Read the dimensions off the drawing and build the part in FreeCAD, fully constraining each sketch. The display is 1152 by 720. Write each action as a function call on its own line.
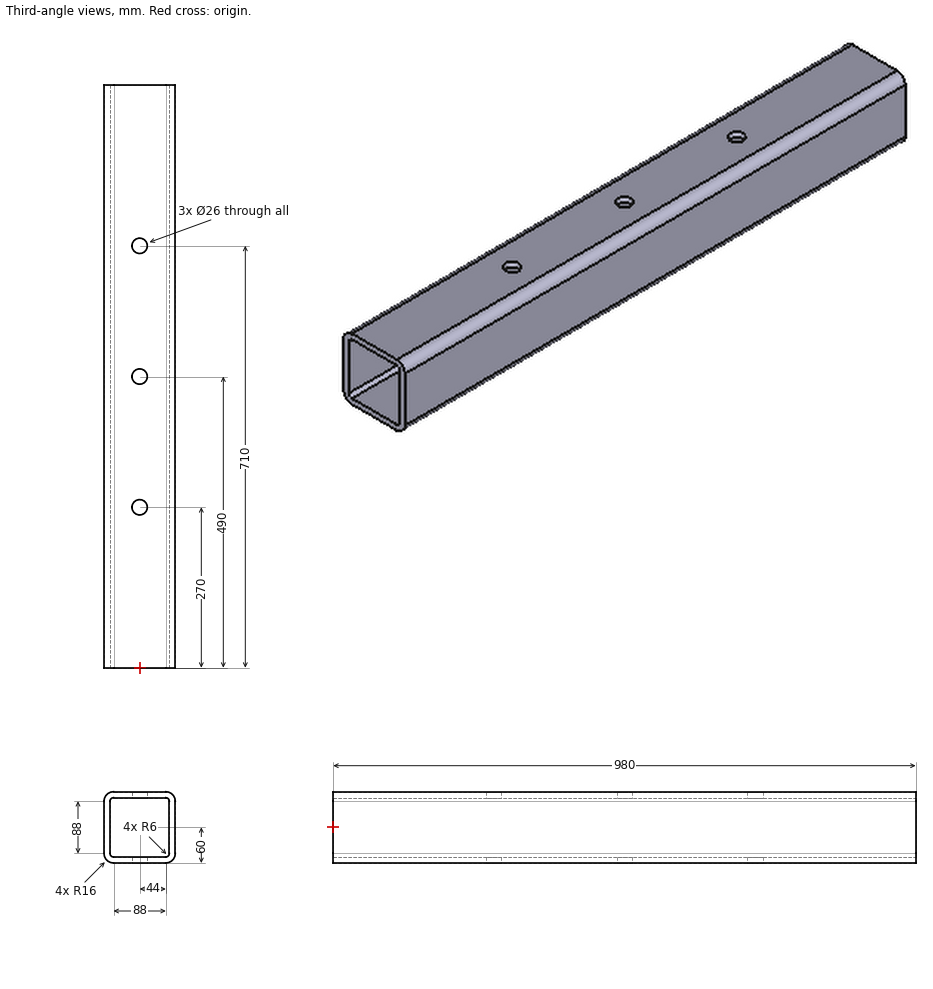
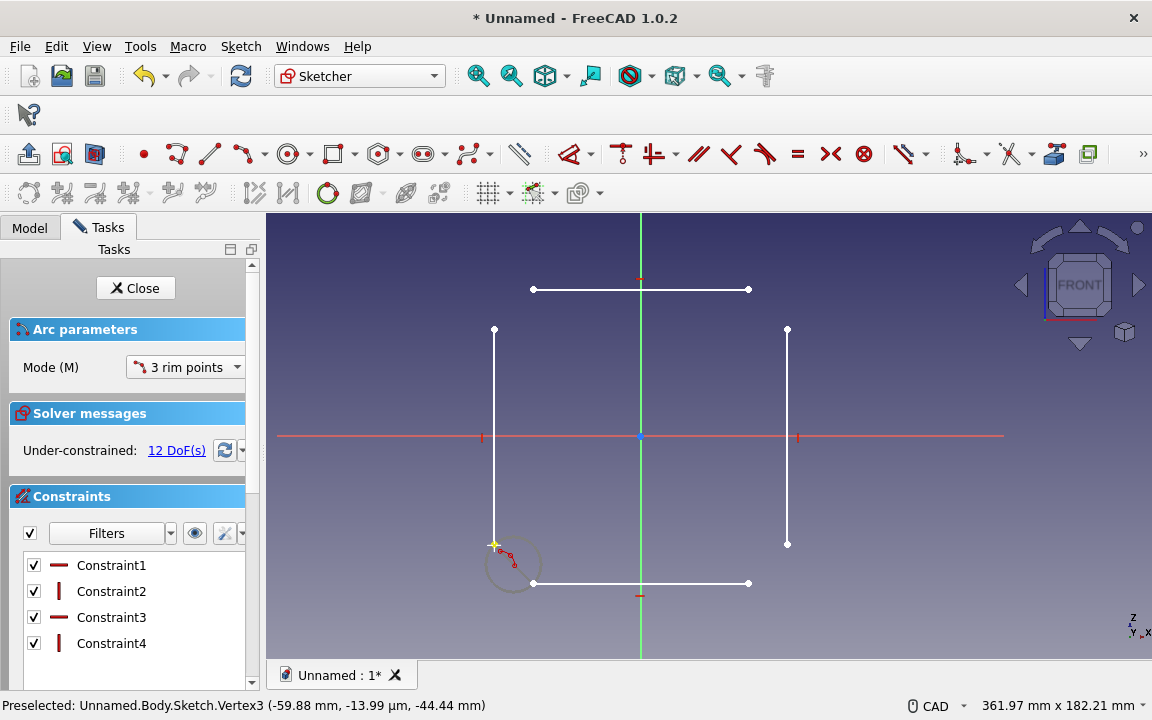
scroll(505, 572, up, 2)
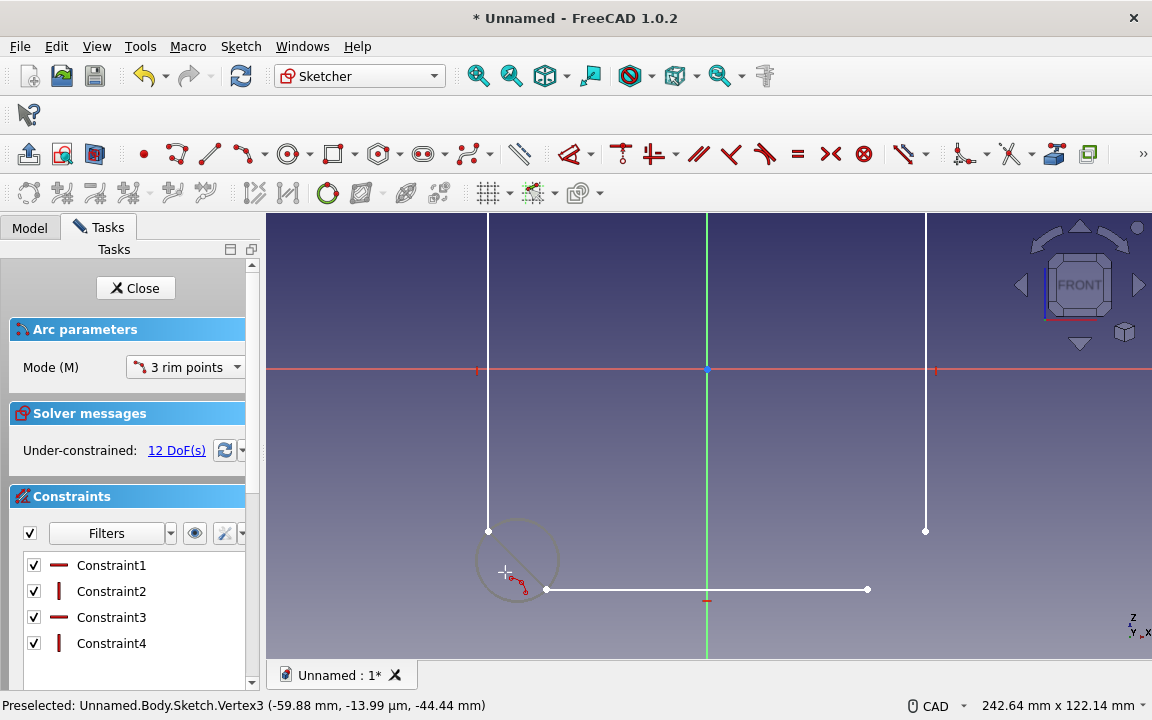
click(505, 571)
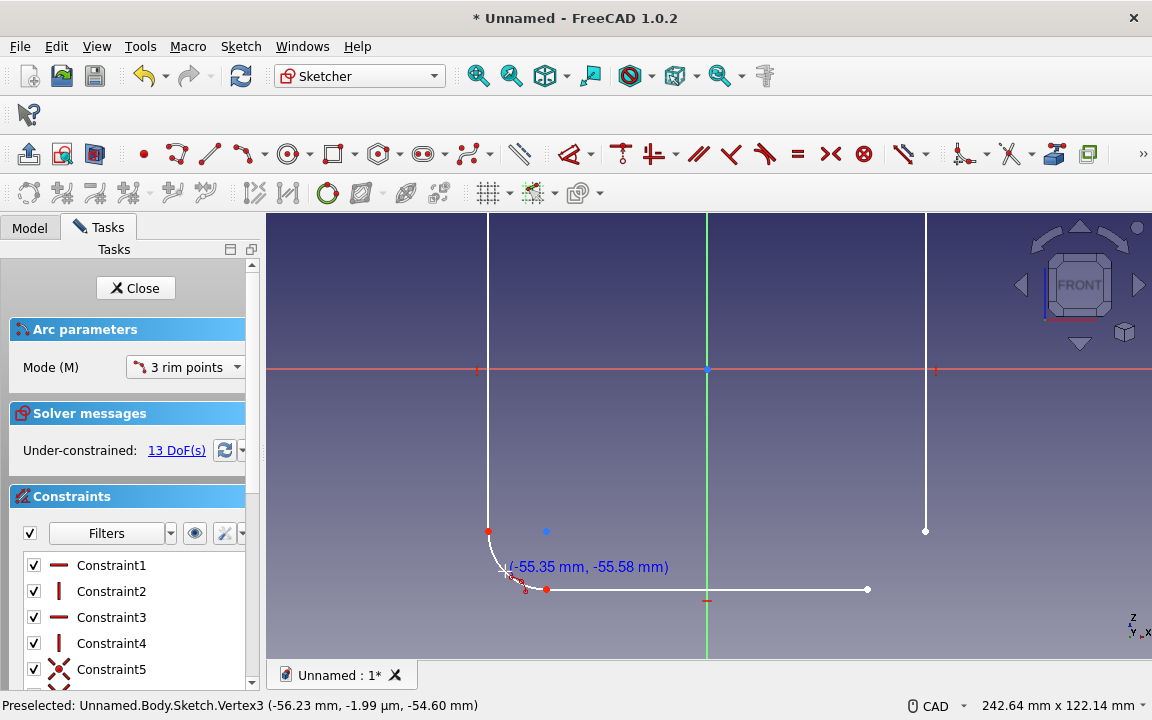
scroll(505, 572, down, 2)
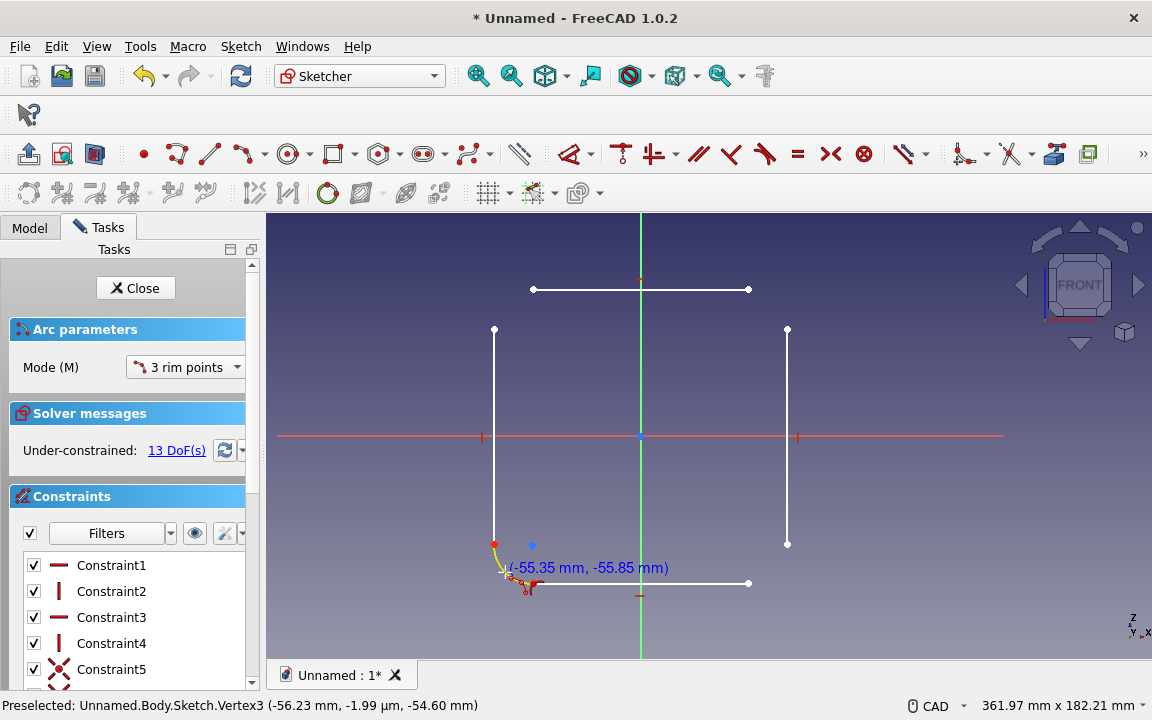
click(494, 330)
click(533, 290)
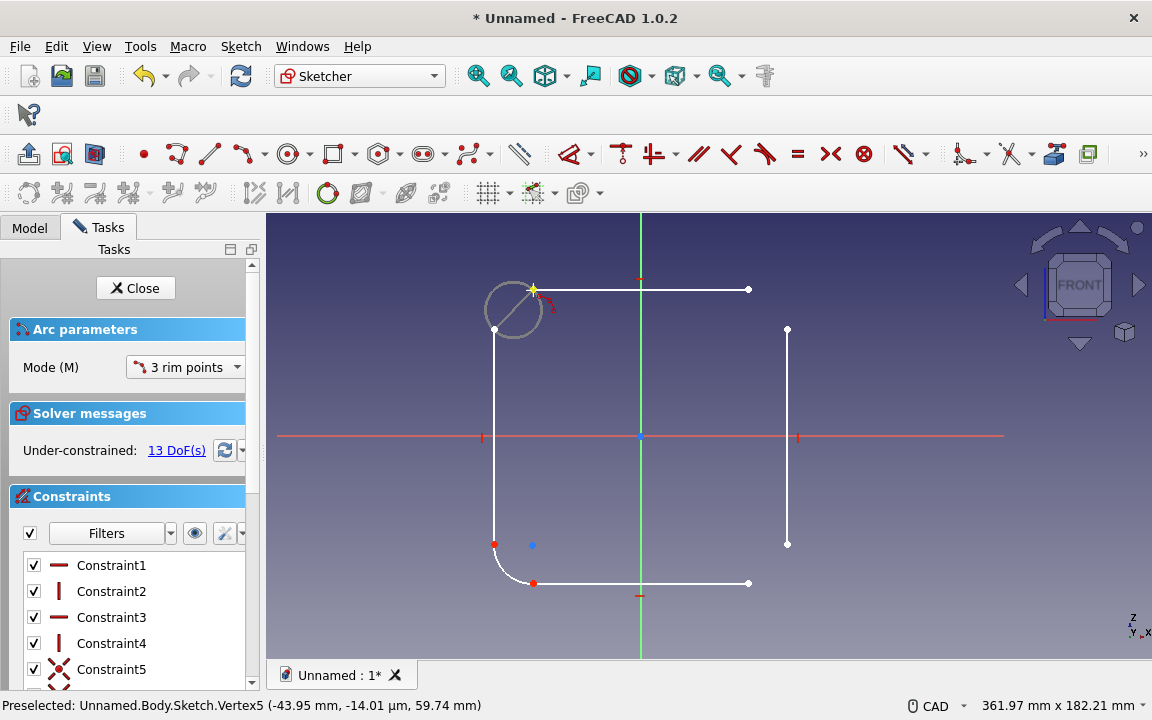
scroll(505, 301, up, 2)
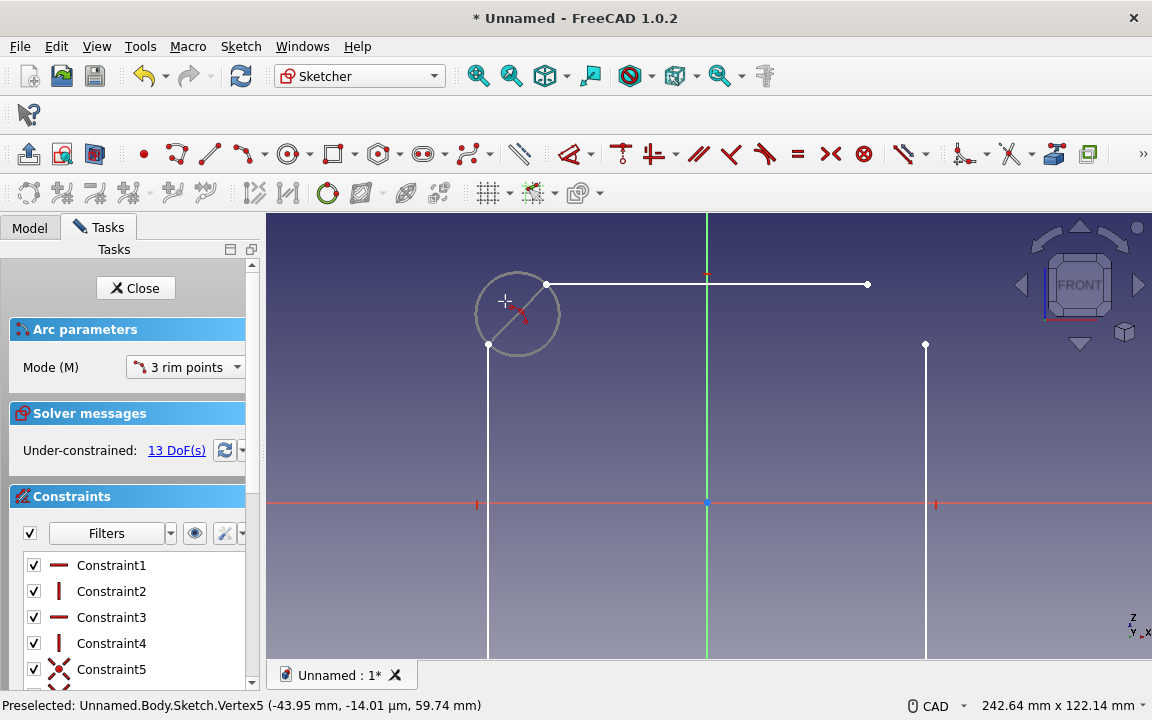
click(505, 301)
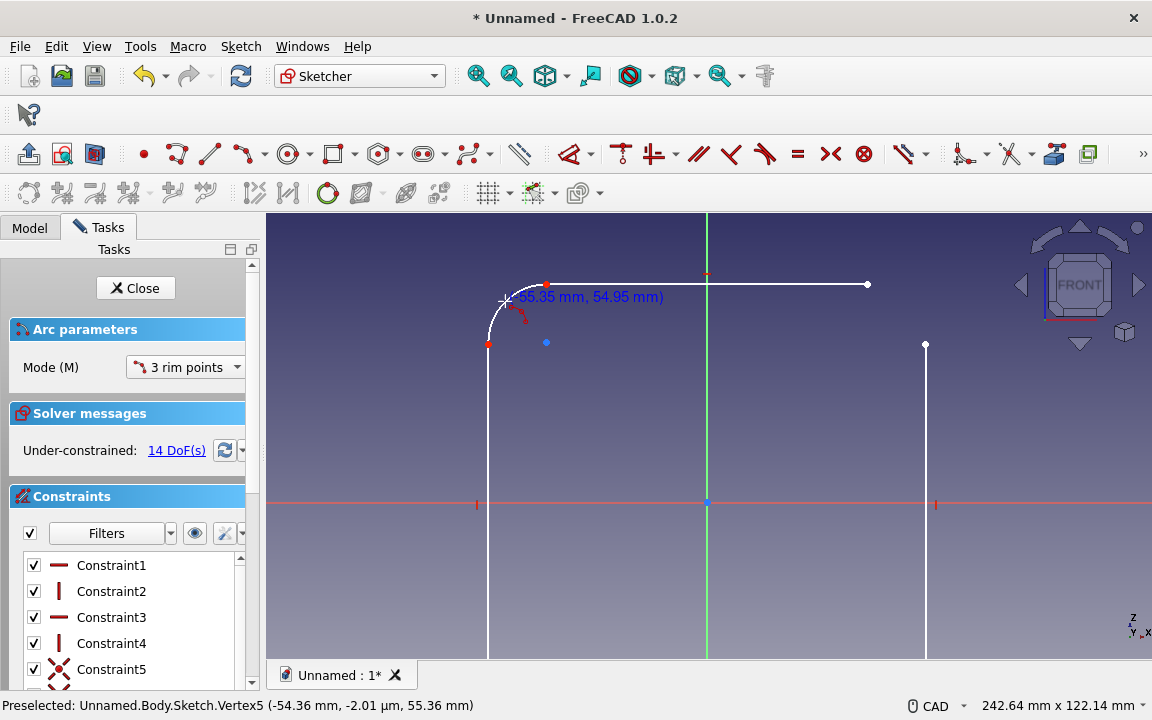
click(867, 284)
click(926, 344)
click(909, 301)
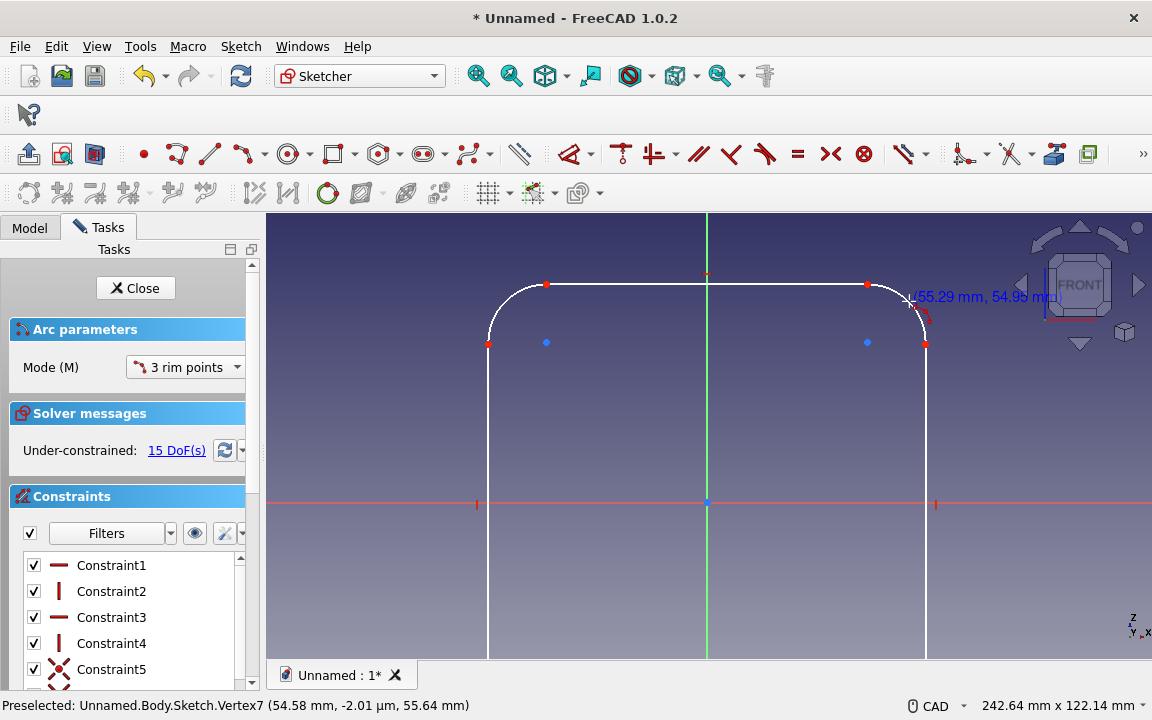
scroll(505, 301, down, 2)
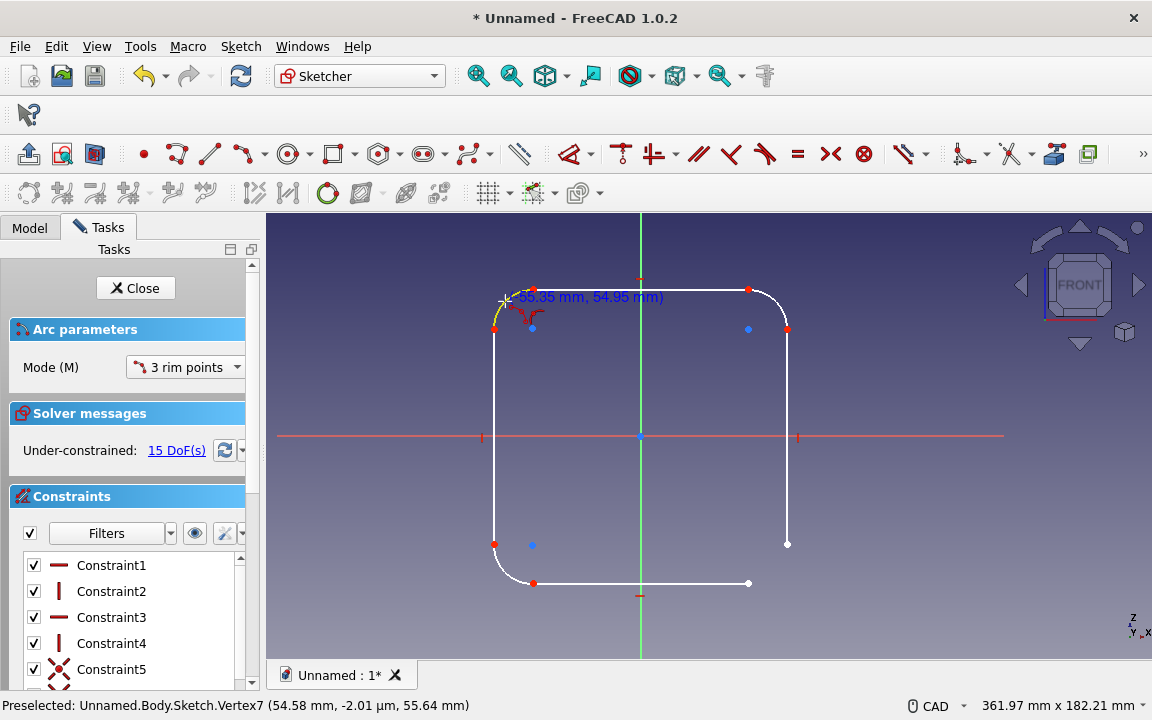
click(787, 545)
click(748, 584)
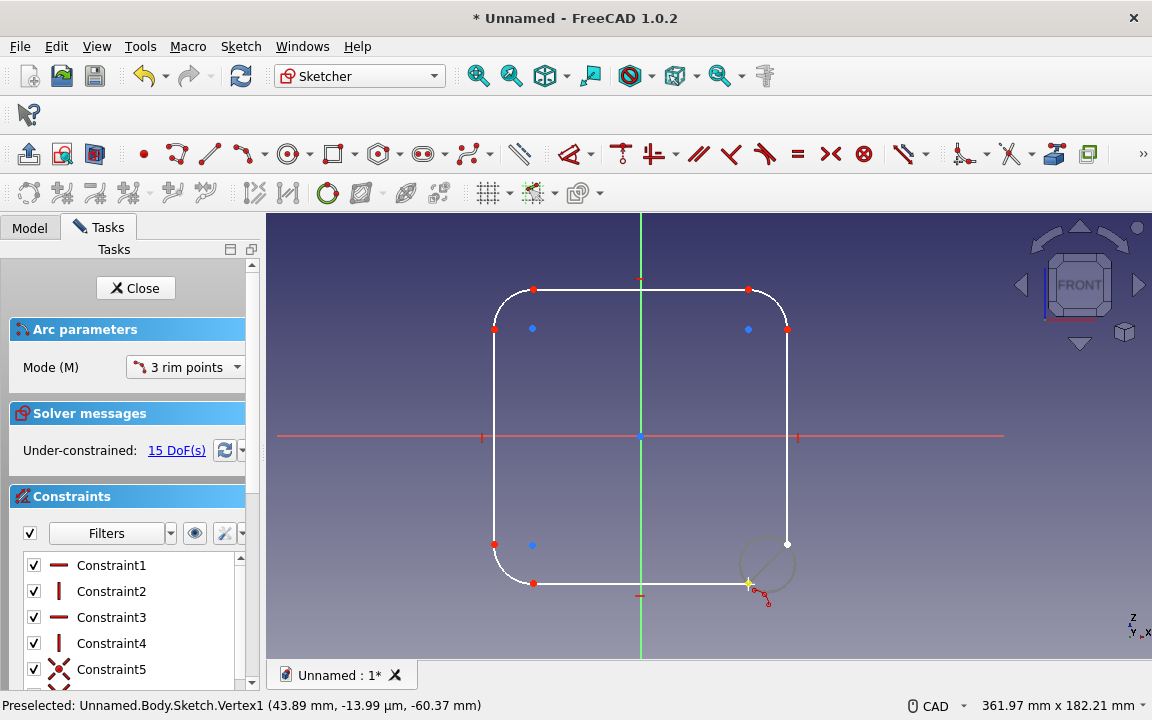
scroll(776, 572, up, 2)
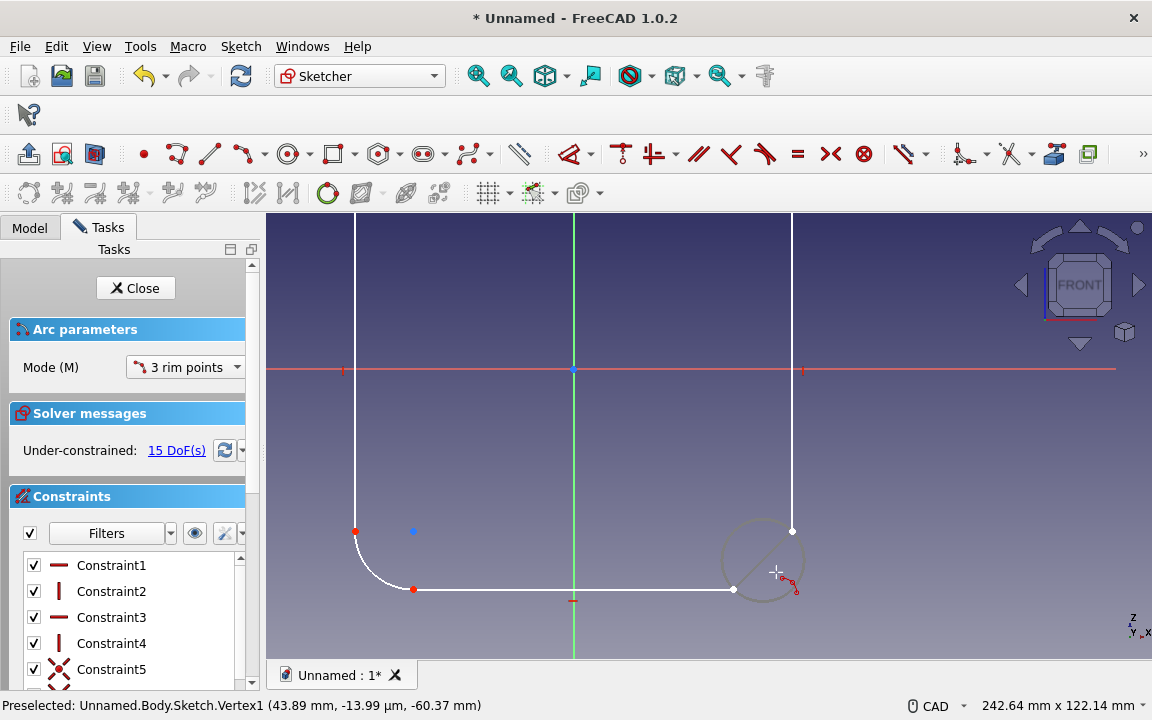
click(776, 571)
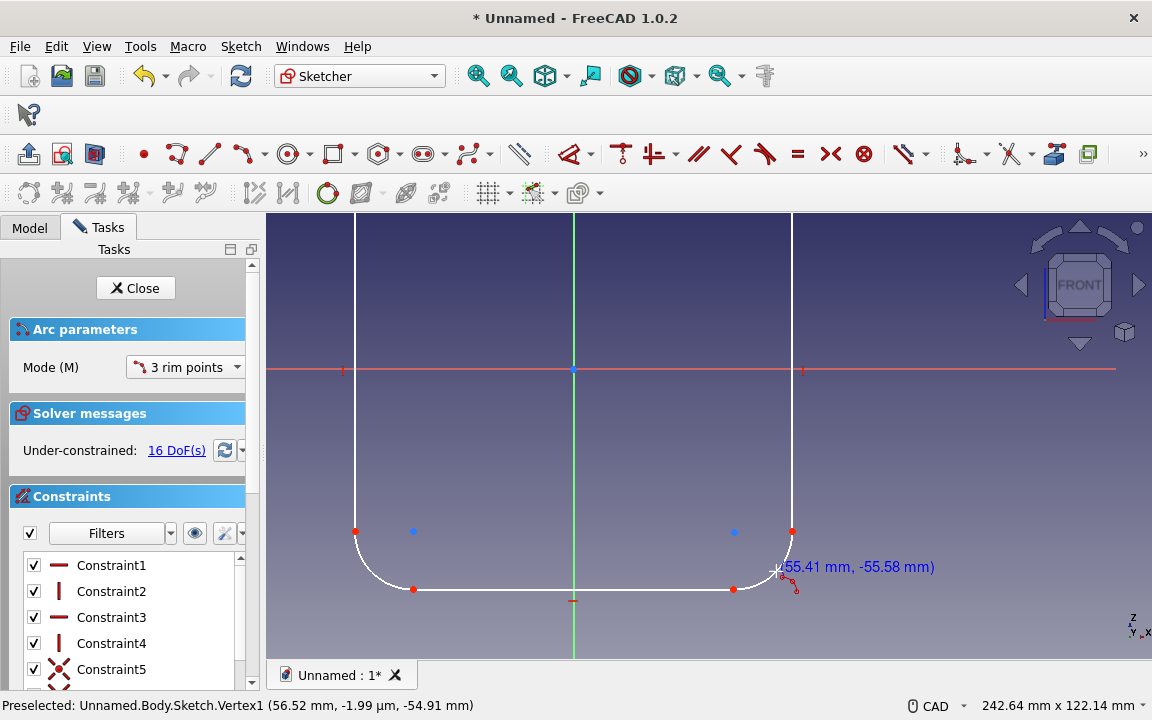
click(210, 154)